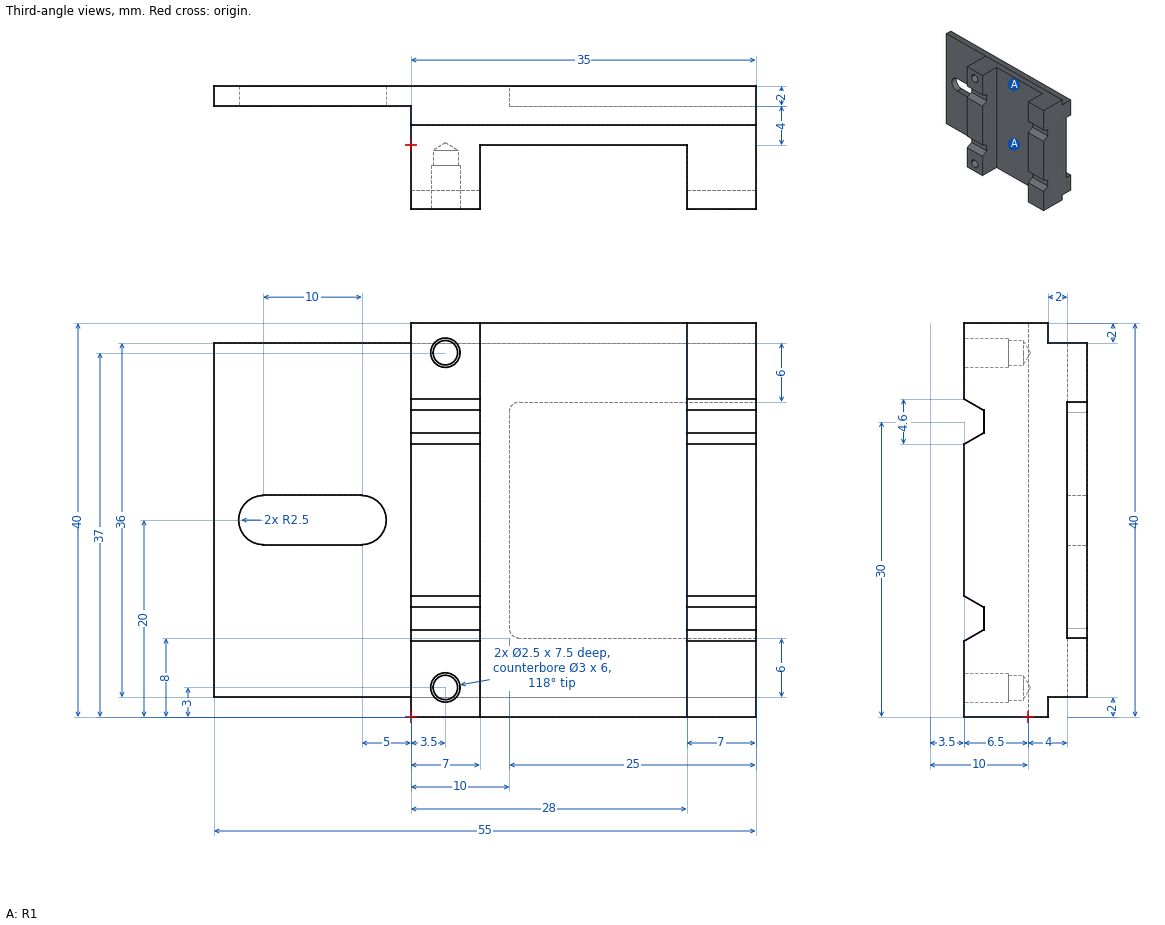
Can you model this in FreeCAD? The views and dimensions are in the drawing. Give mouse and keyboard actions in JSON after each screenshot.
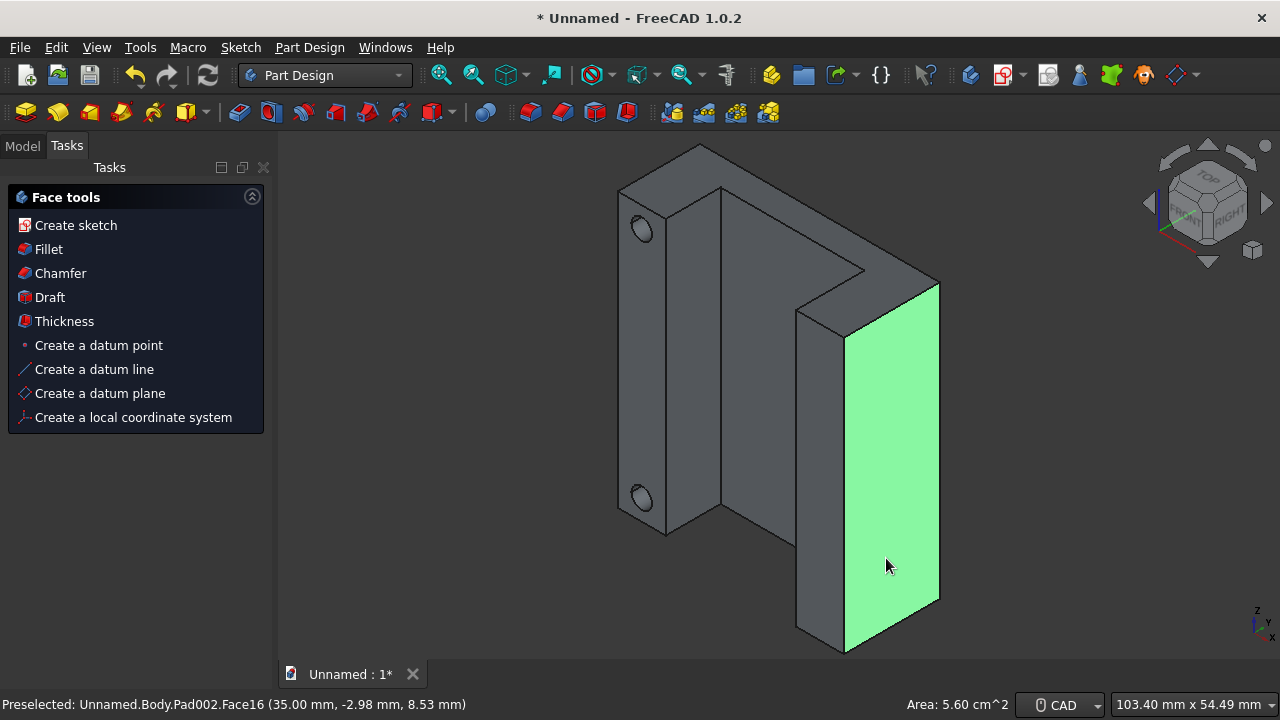
{"action": "left_click", "coordinate": [1004, 76]}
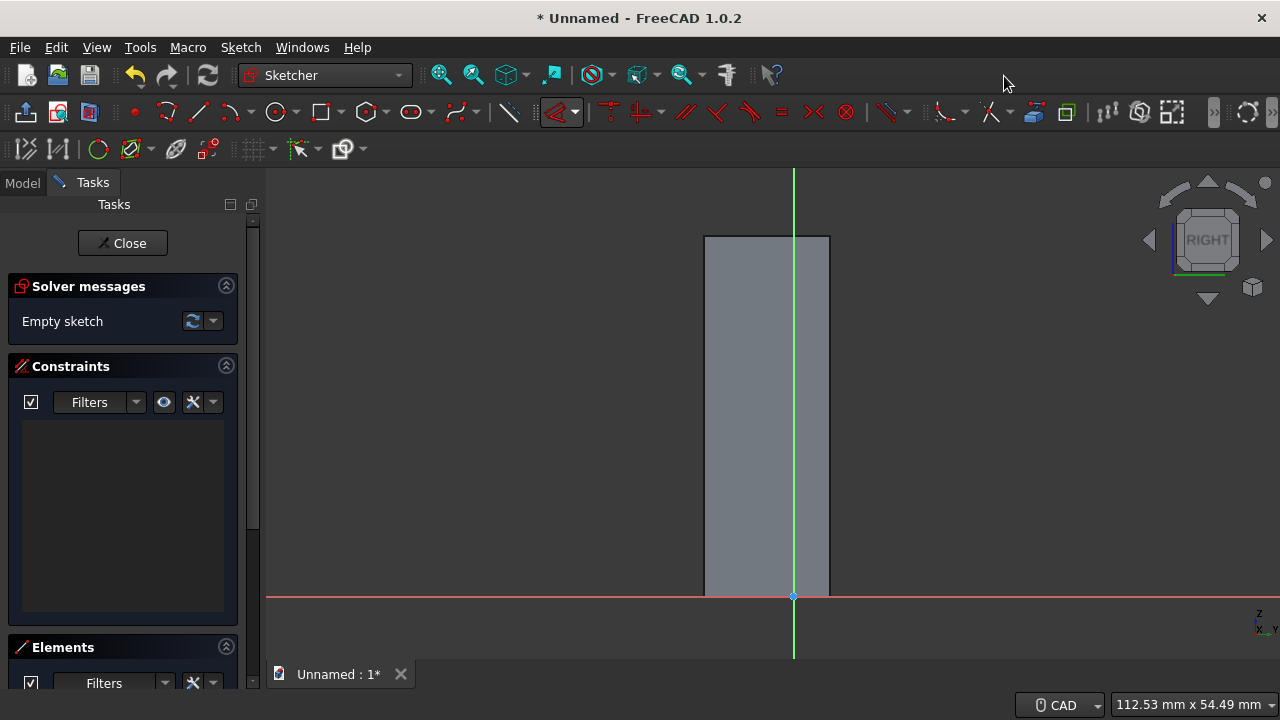
{"action": "left_click", "coordinate": [322, 112]}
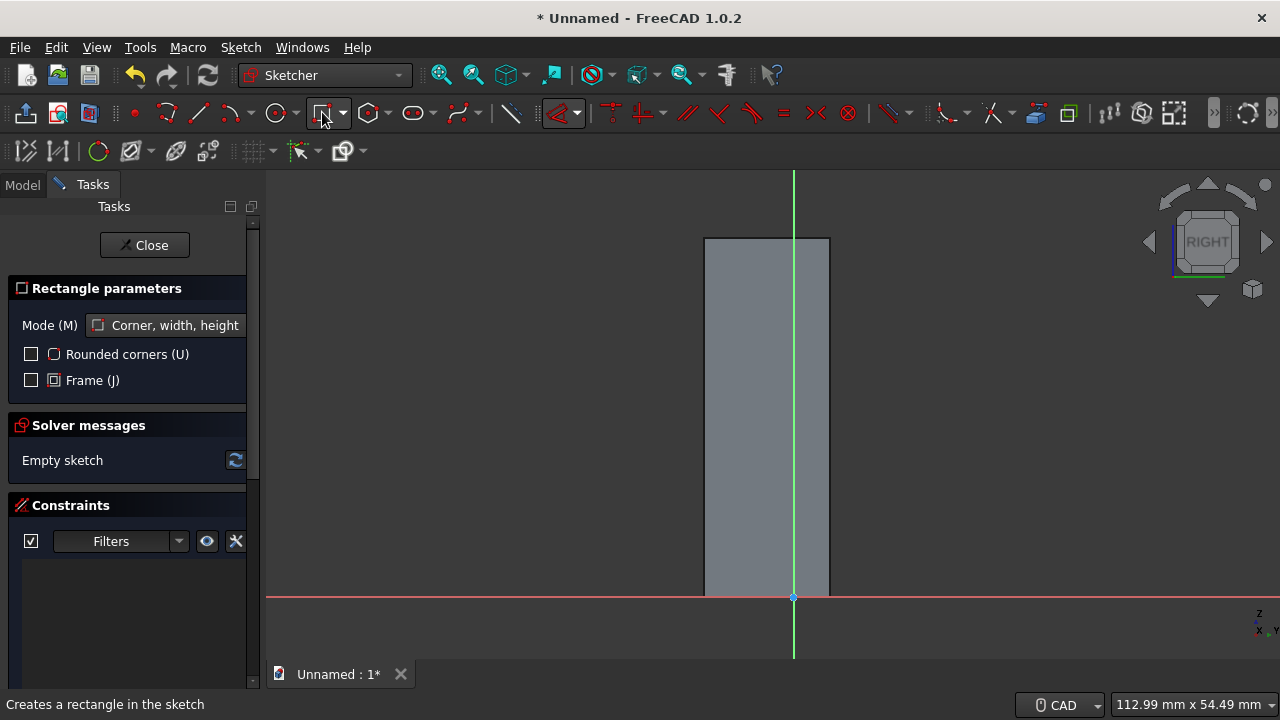
{"action": "left_click", "coordinate": [704, 238]}
{"action": "left_click", "coordinate": [735, 597]}
{"action": "key", "text": "Escape"}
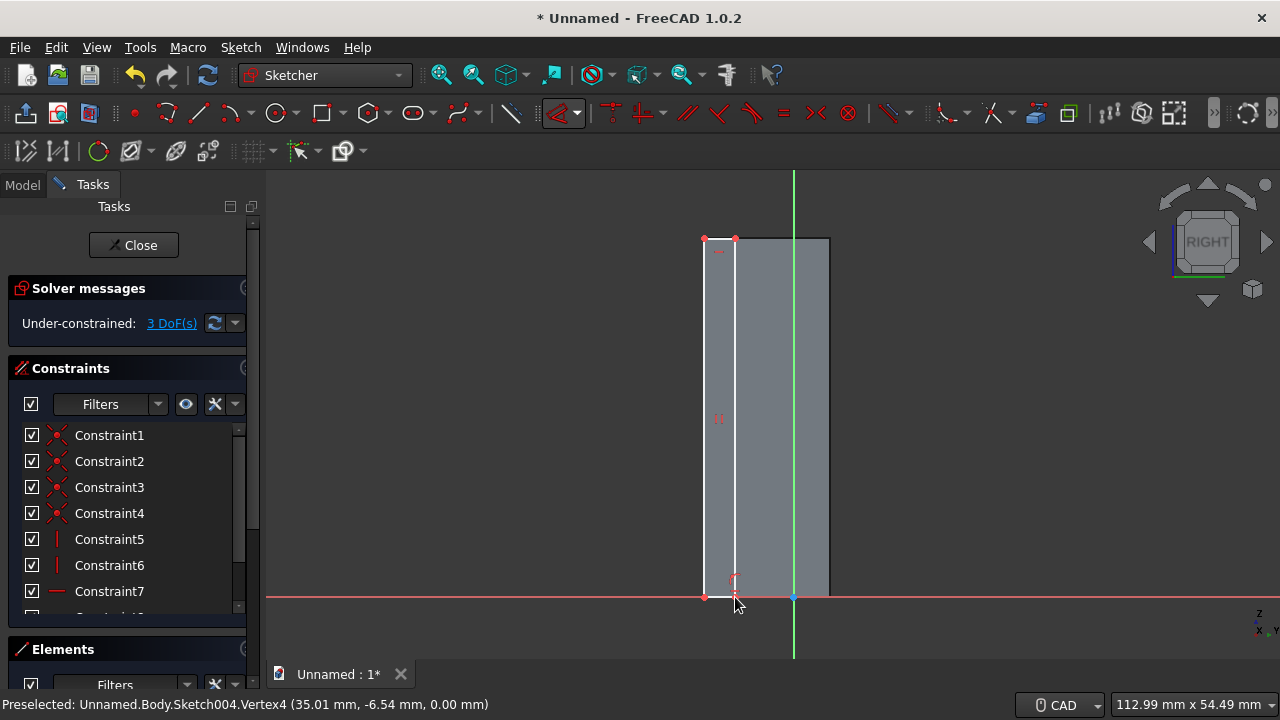
{"action": "left_click", "coordinate": [704, 346]}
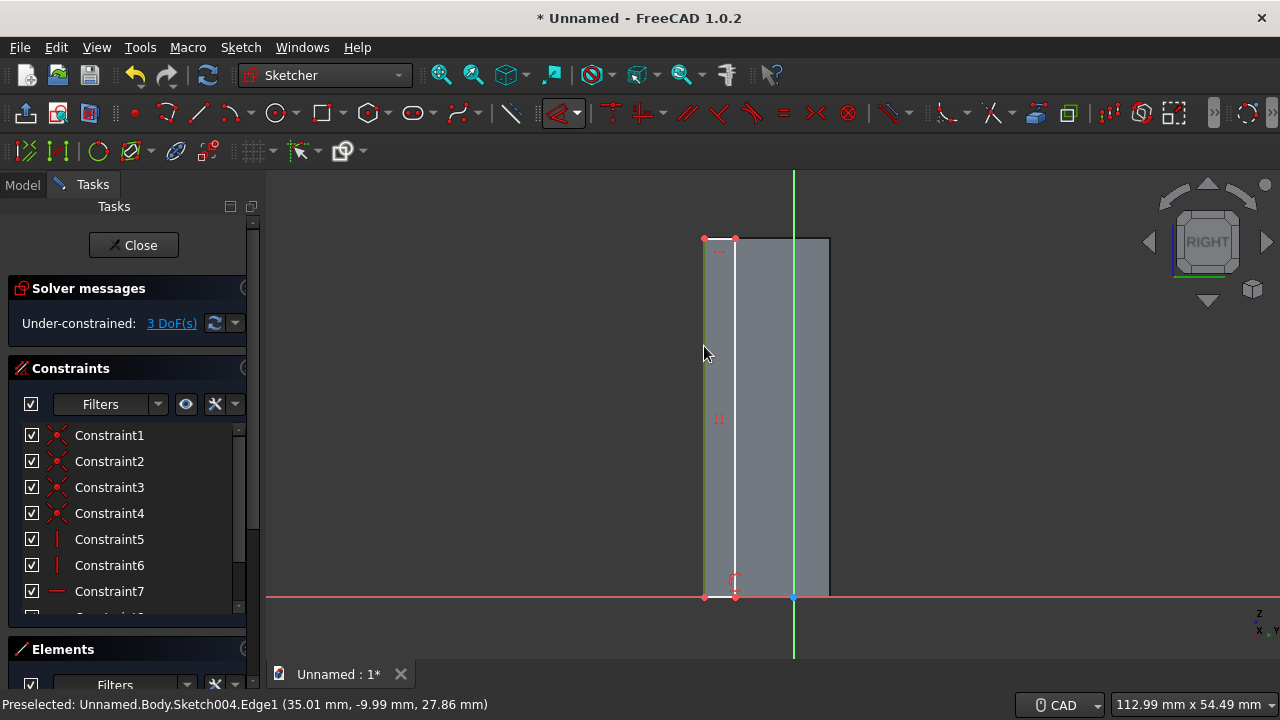
{"action": "left_click", "coordinate": [580, 114]}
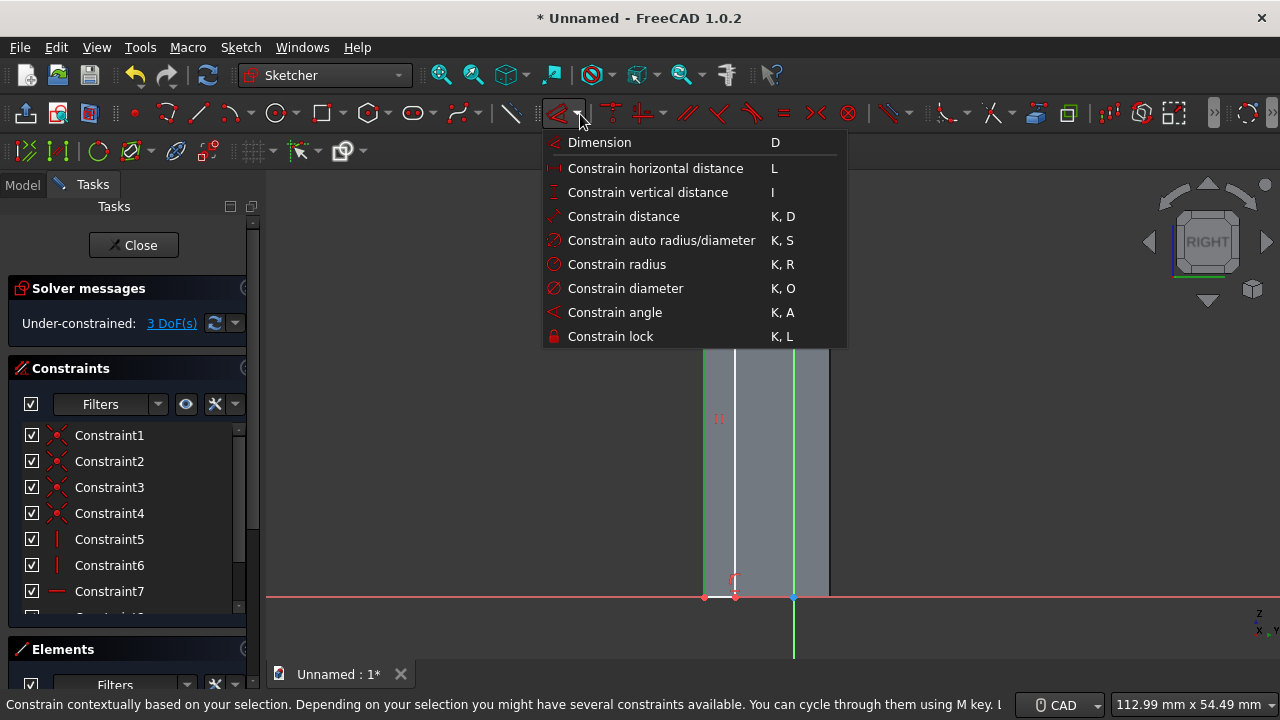
{"action": "left_click", "coordinate": [695, 192]}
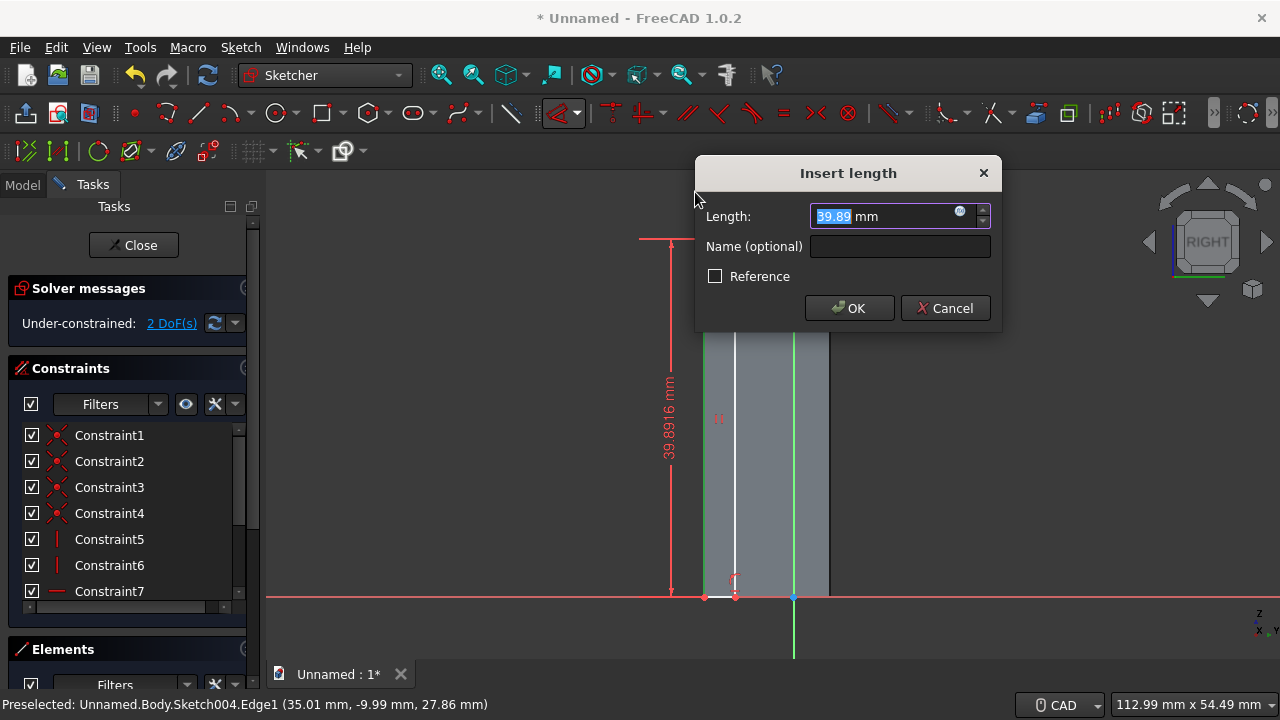
{"action": "type", "text": "40"}
{"action": "key", "text": "Return"}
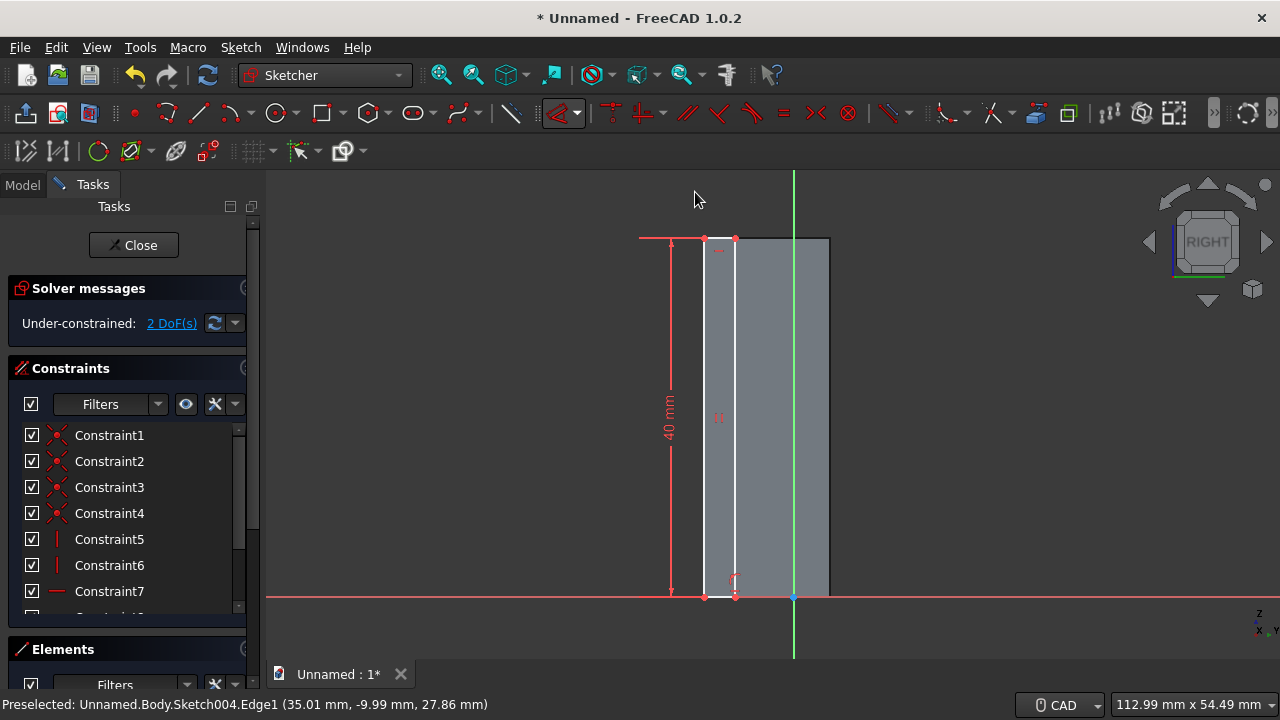
{"action": "scroll", "coordinate": [713, 597], "scroll_direction": "up", "scroll_amount": 2}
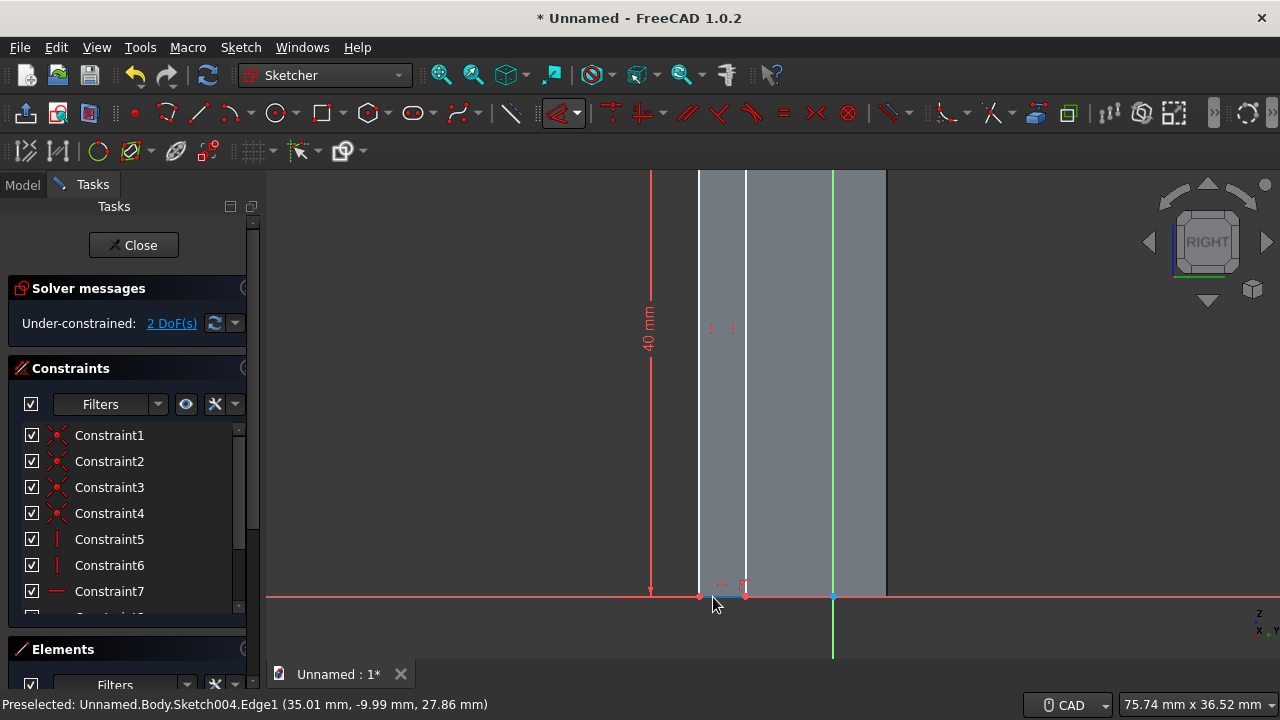
{"action": "left_click", "coordinate": [713, 597]}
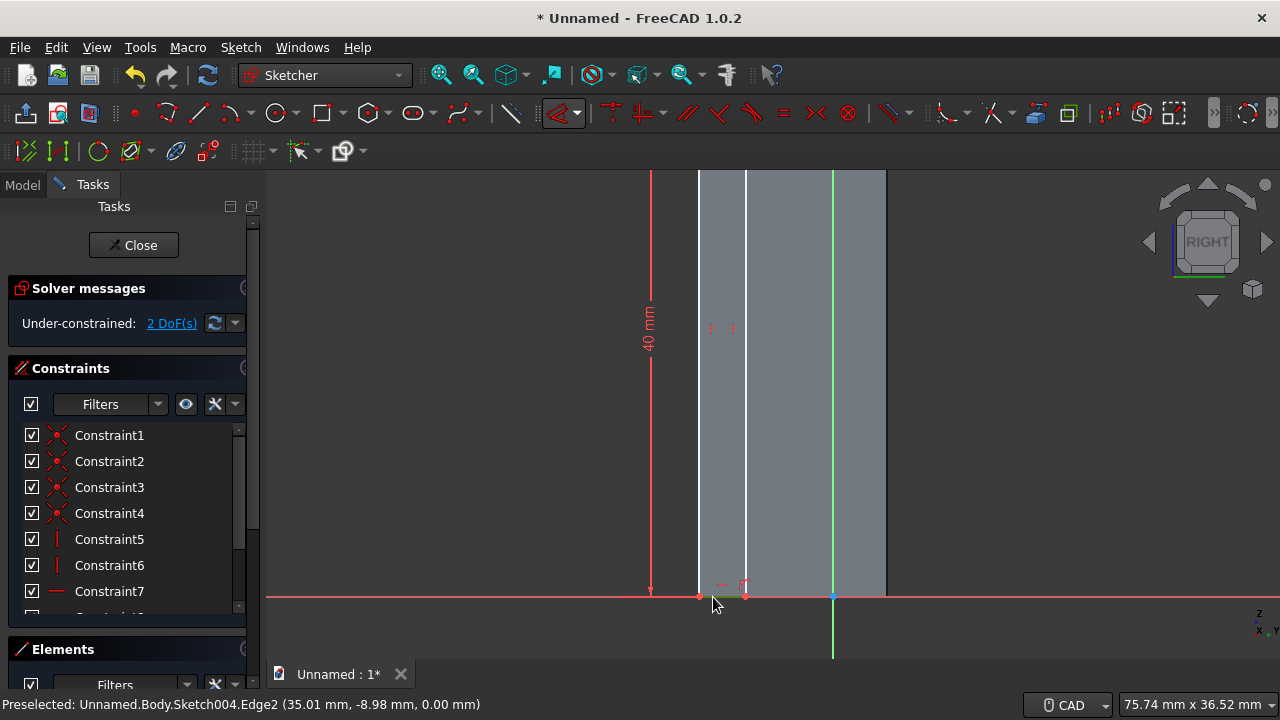
{"action": "left_click", "coordinate": [580, 114]}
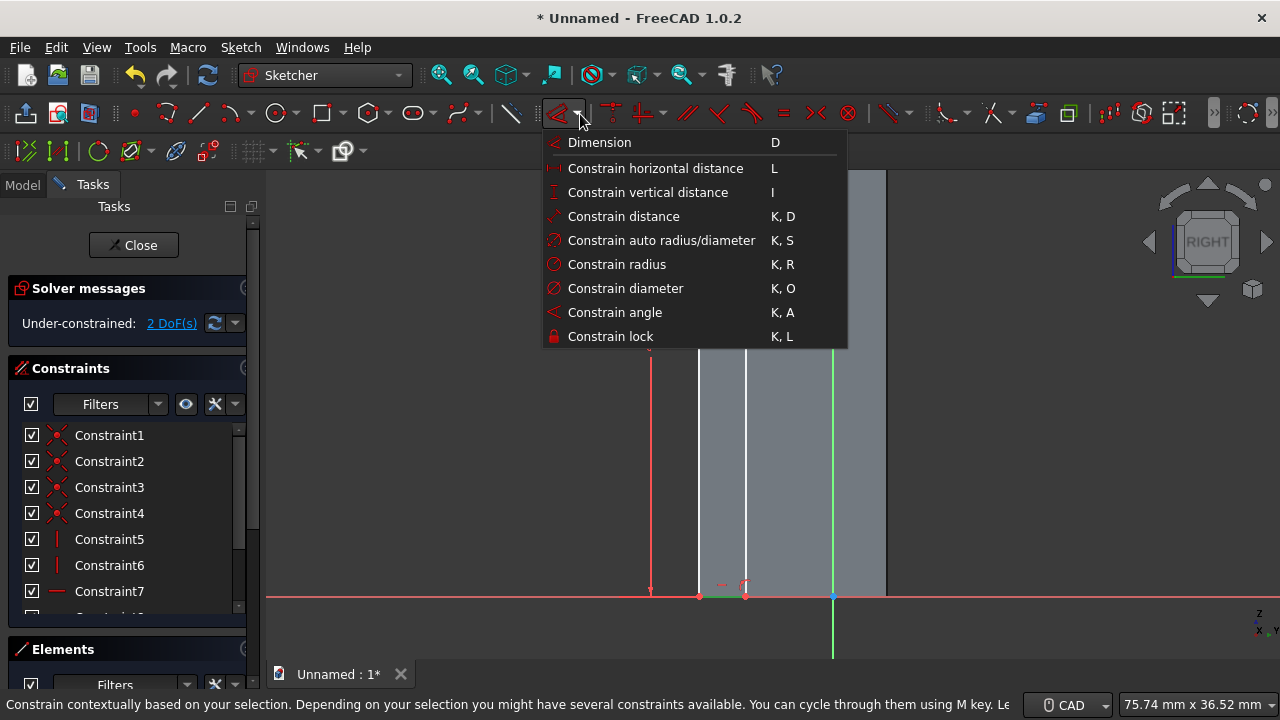
{"action": "left_click", "coordinate": [695, 168]}